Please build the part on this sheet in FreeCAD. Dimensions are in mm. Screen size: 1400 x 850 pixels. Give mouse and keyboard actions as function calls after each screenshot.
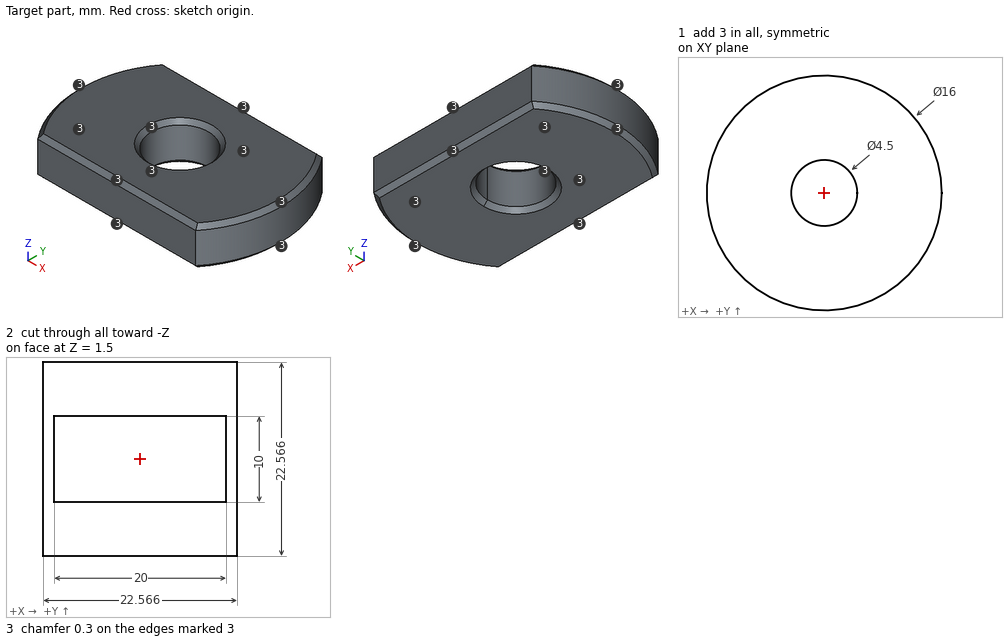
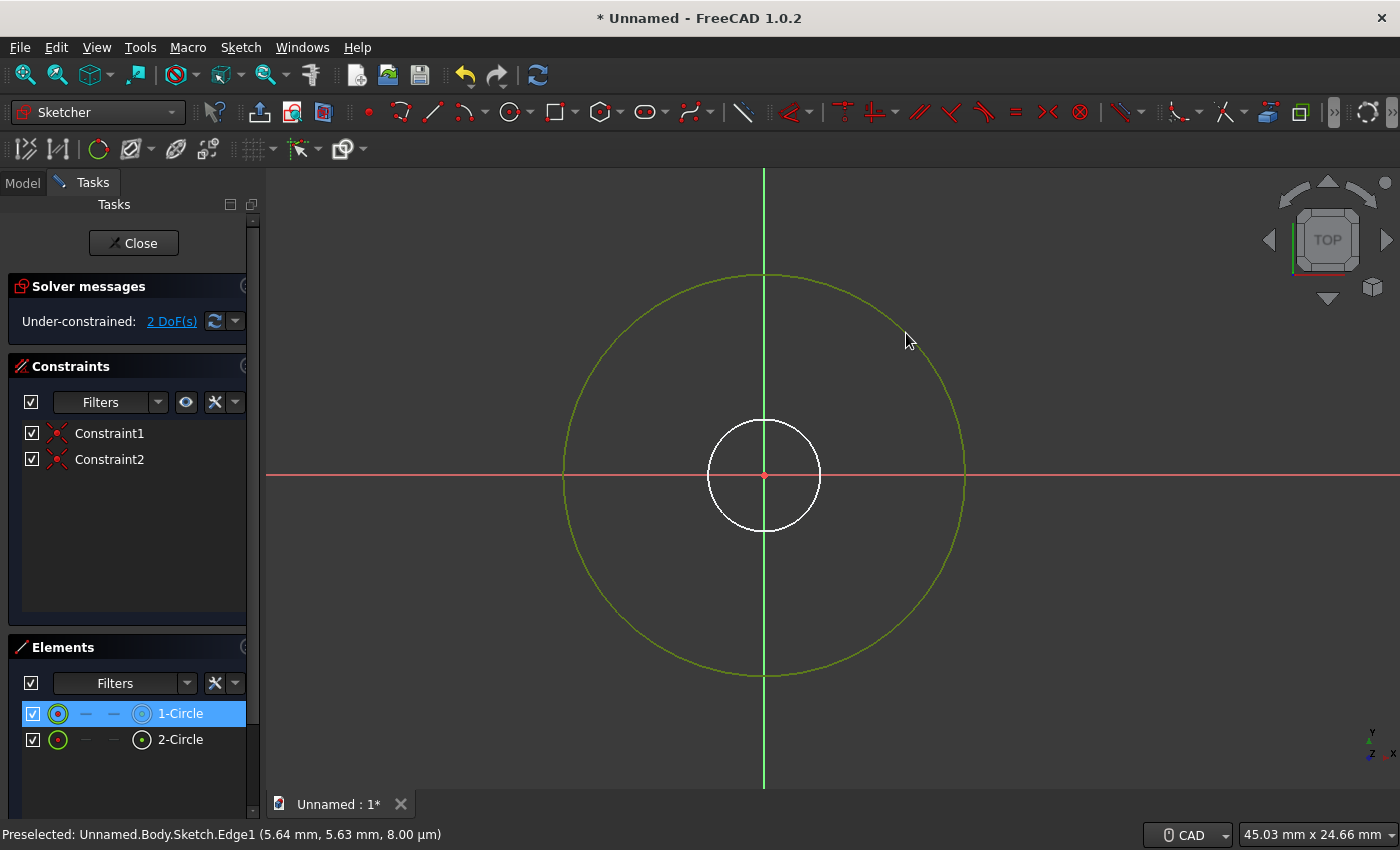
key(k)
key(o)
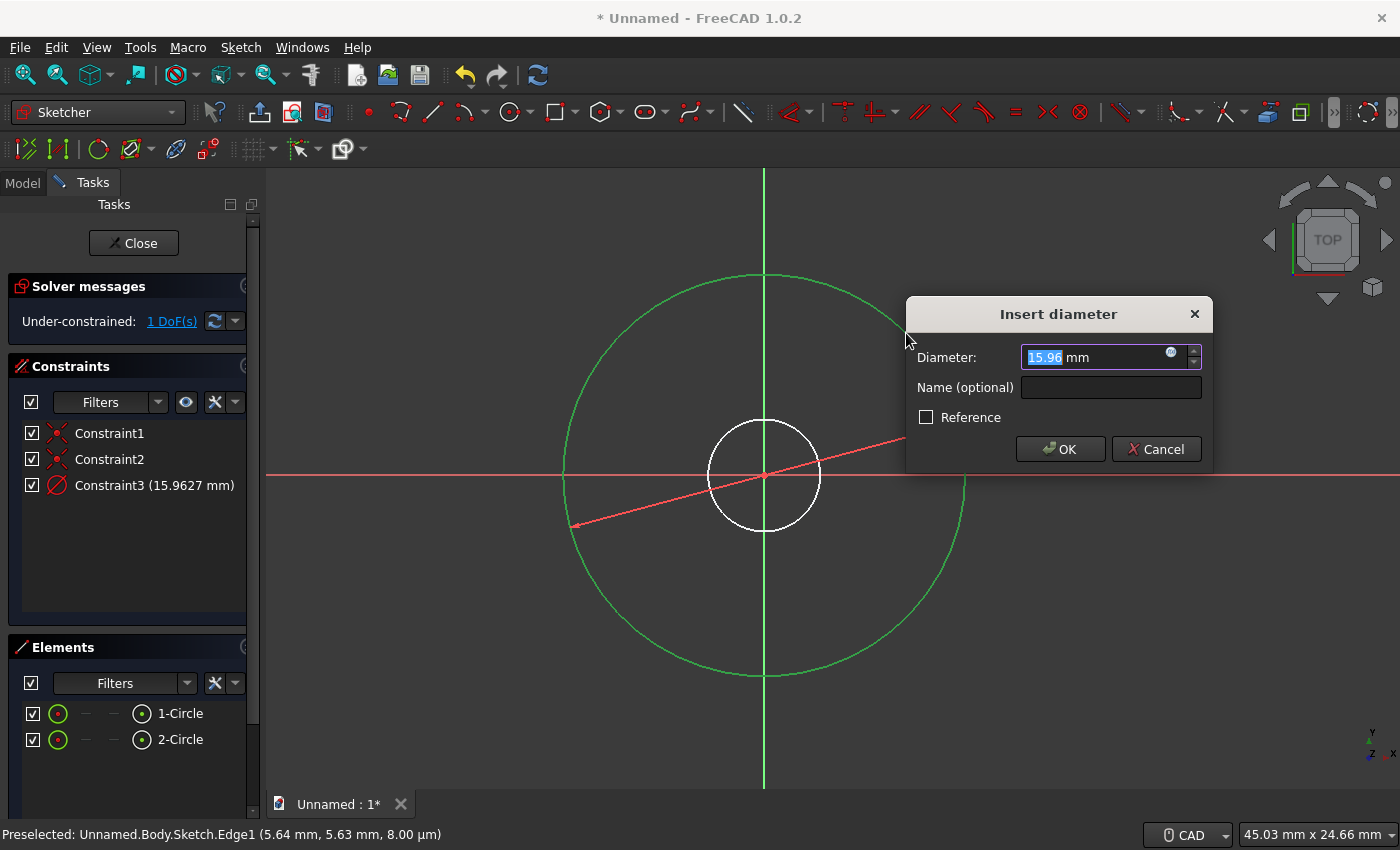
text(16)
key(Return)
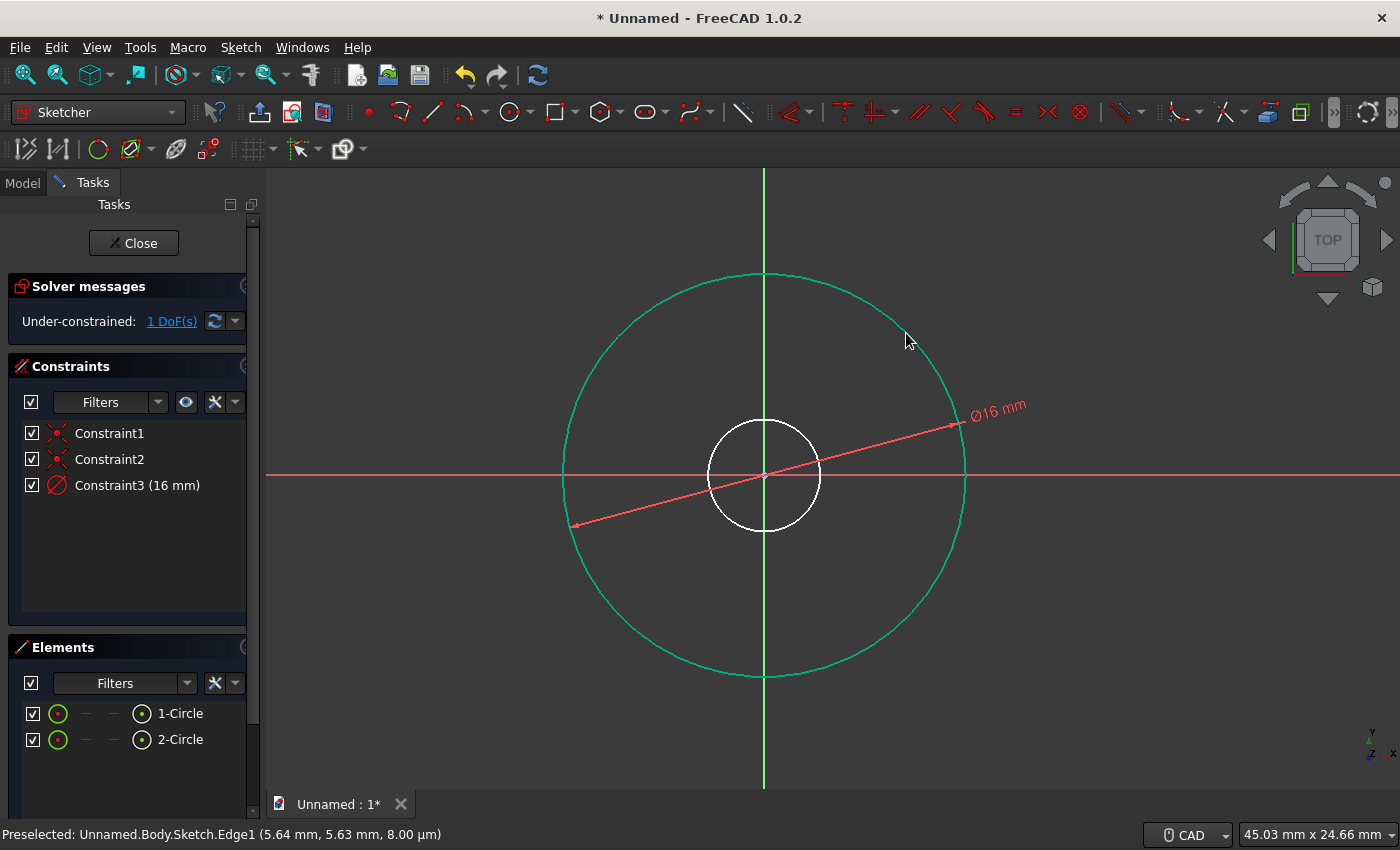
click(804, 436)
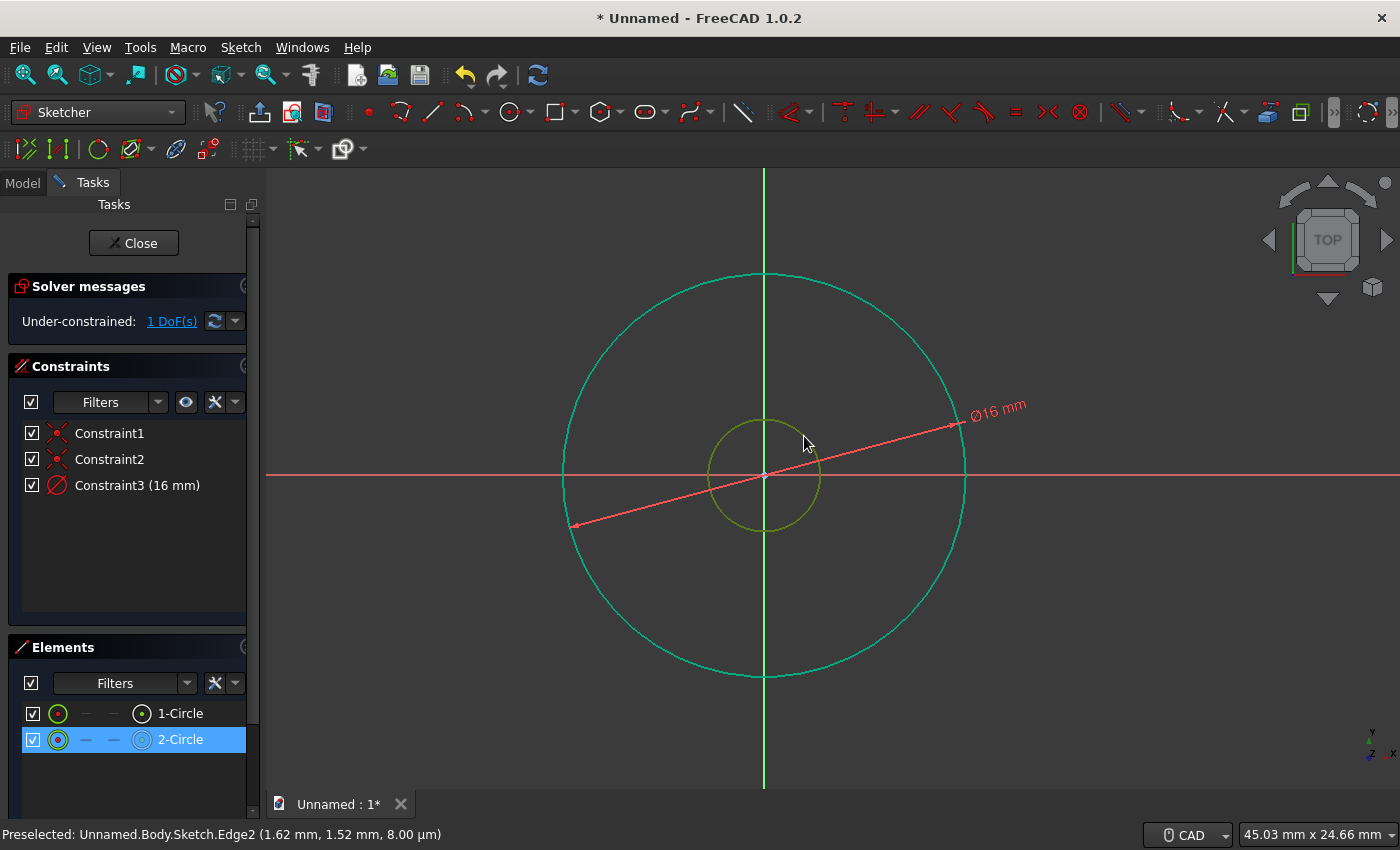
key(k)
key(o)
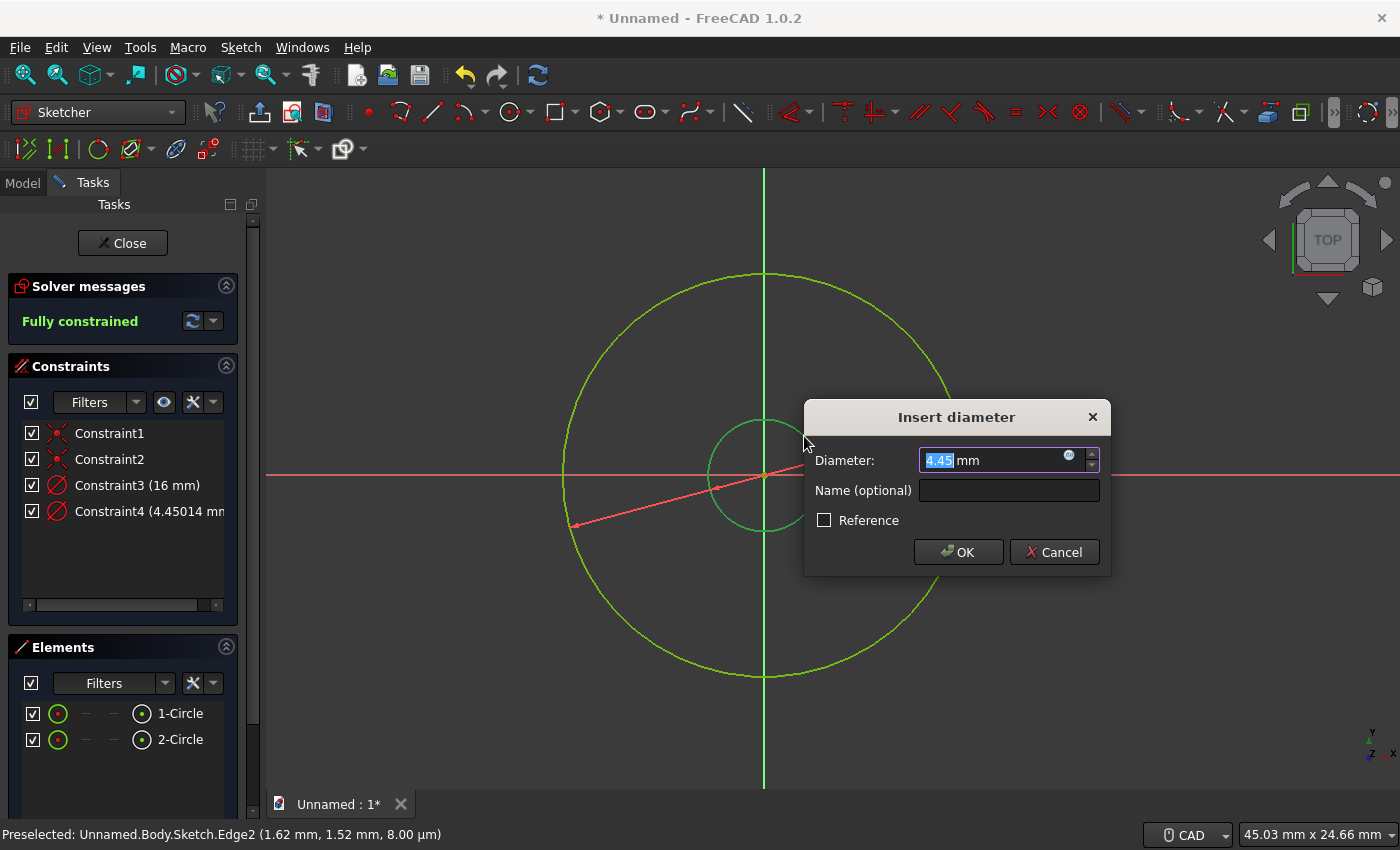
text(4.5)
key(Return)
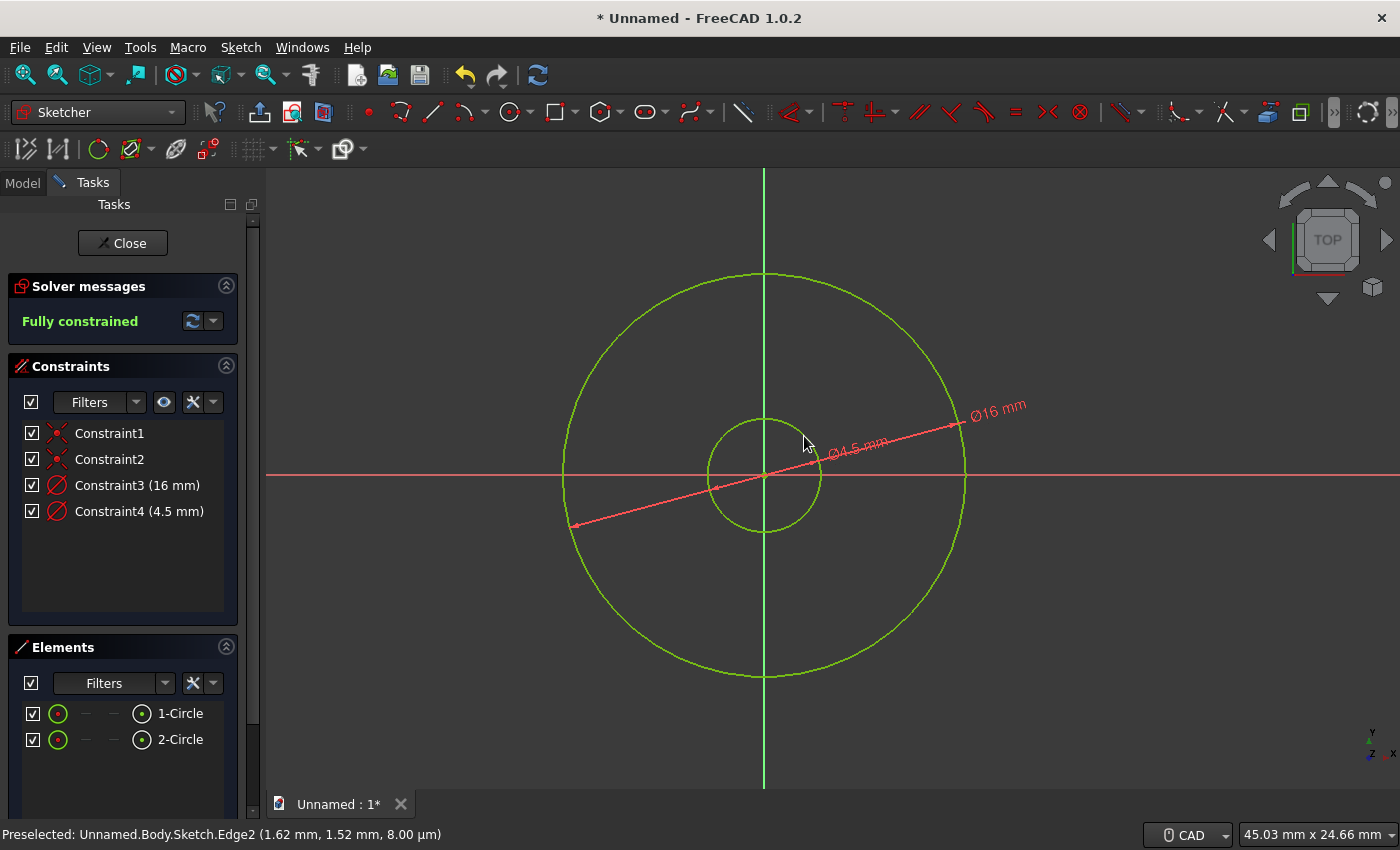
click(123, 243)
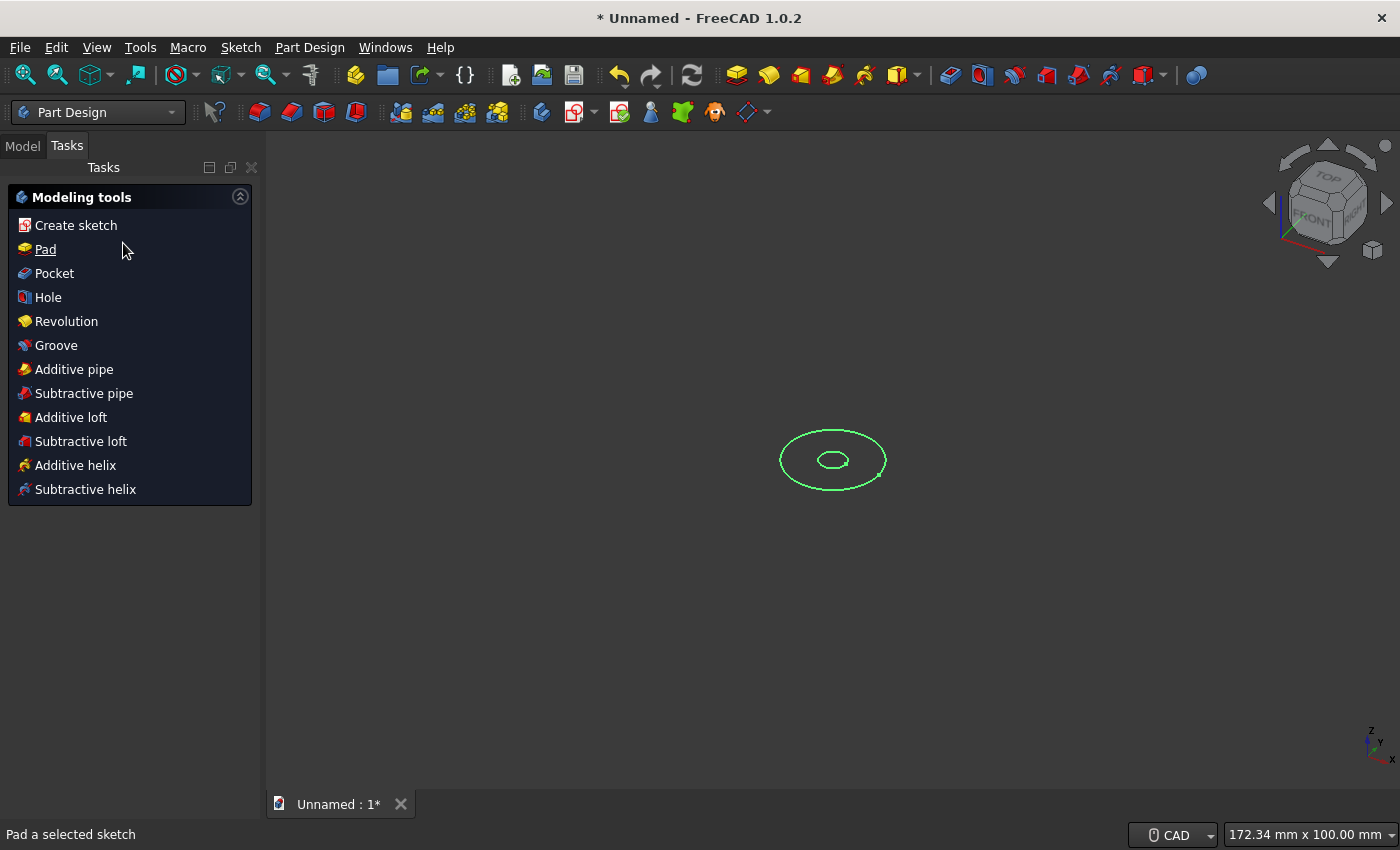
click(738, 76)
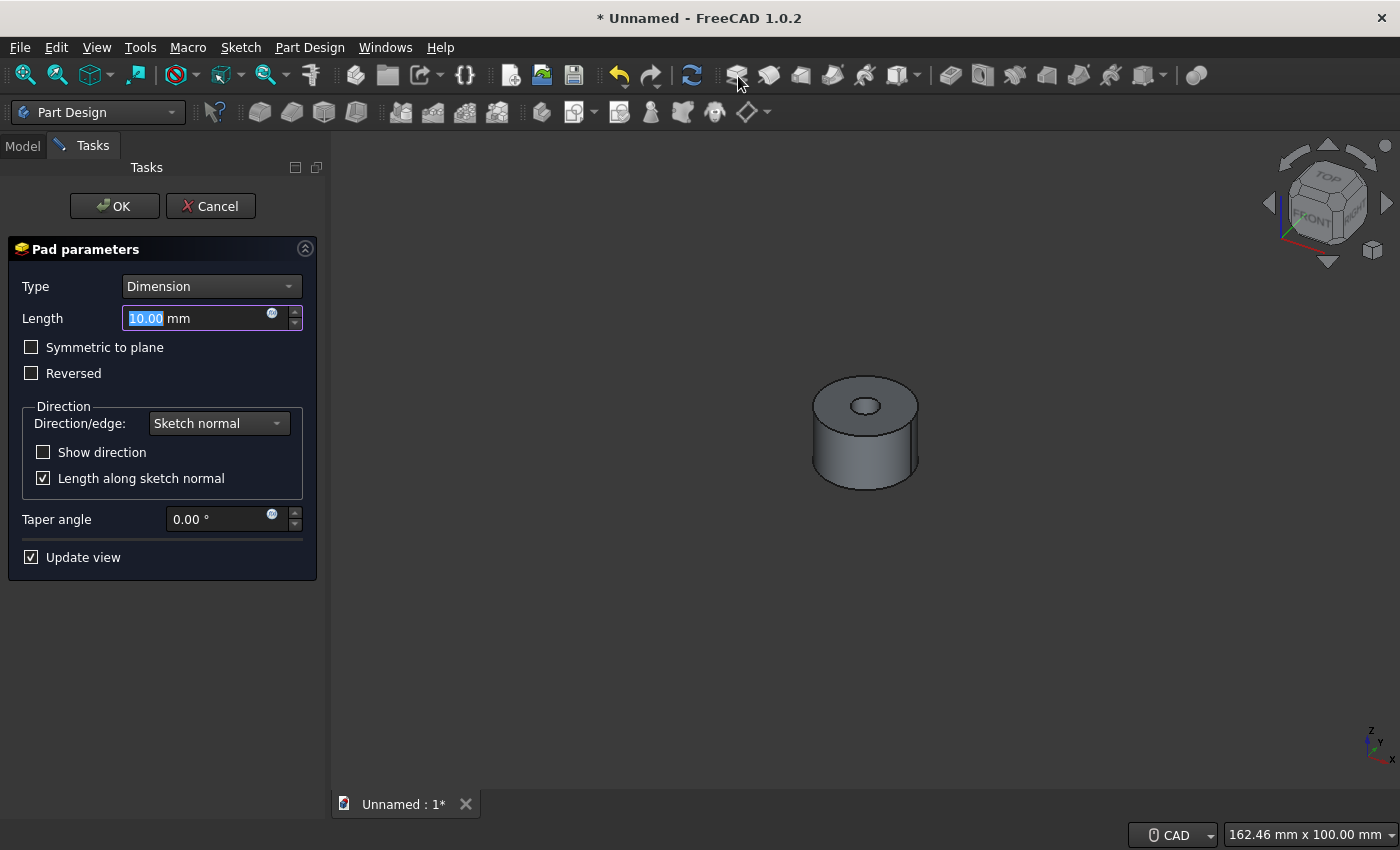
text(3)
key(Tab)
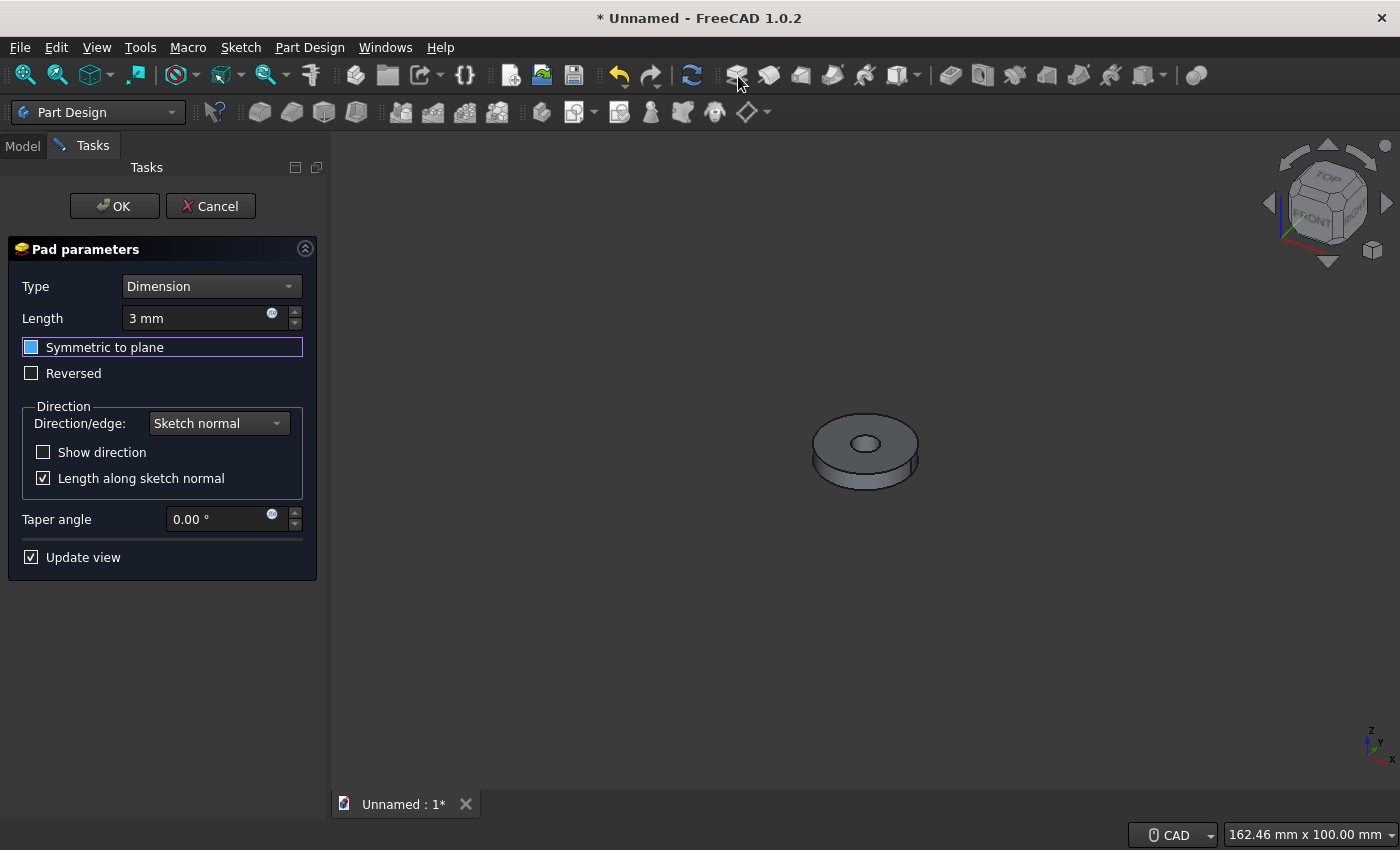
click(30, 347)